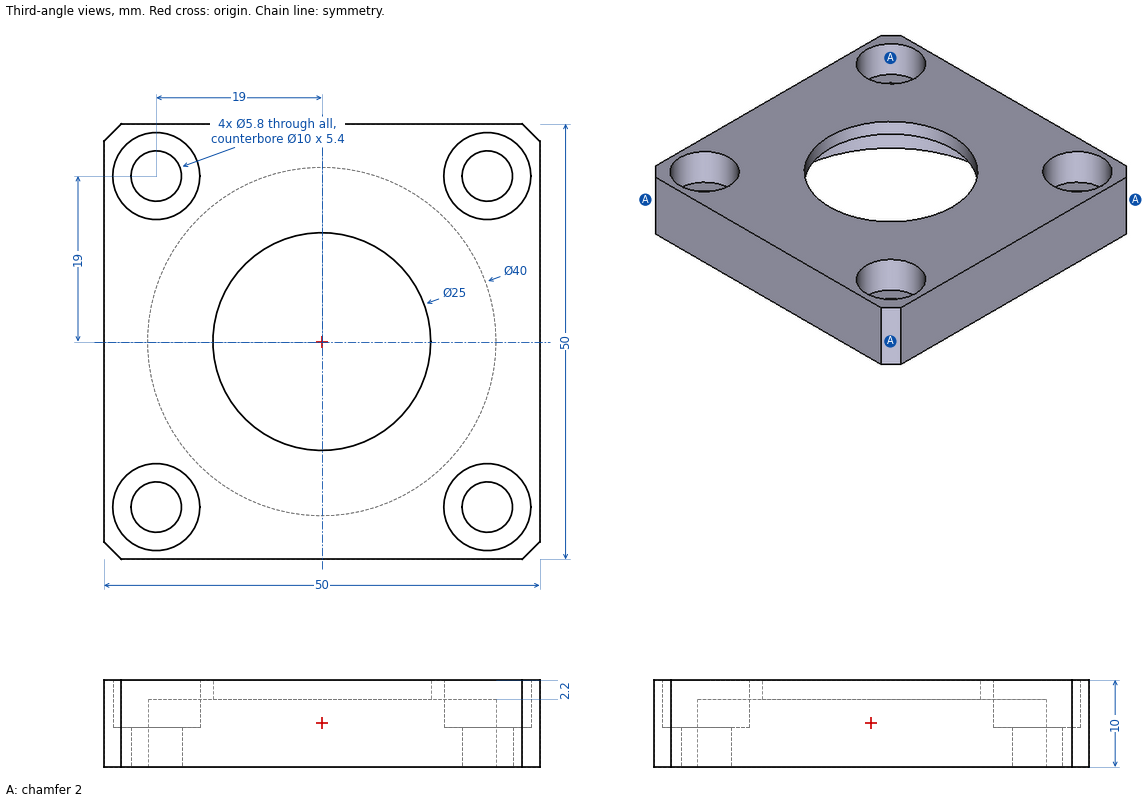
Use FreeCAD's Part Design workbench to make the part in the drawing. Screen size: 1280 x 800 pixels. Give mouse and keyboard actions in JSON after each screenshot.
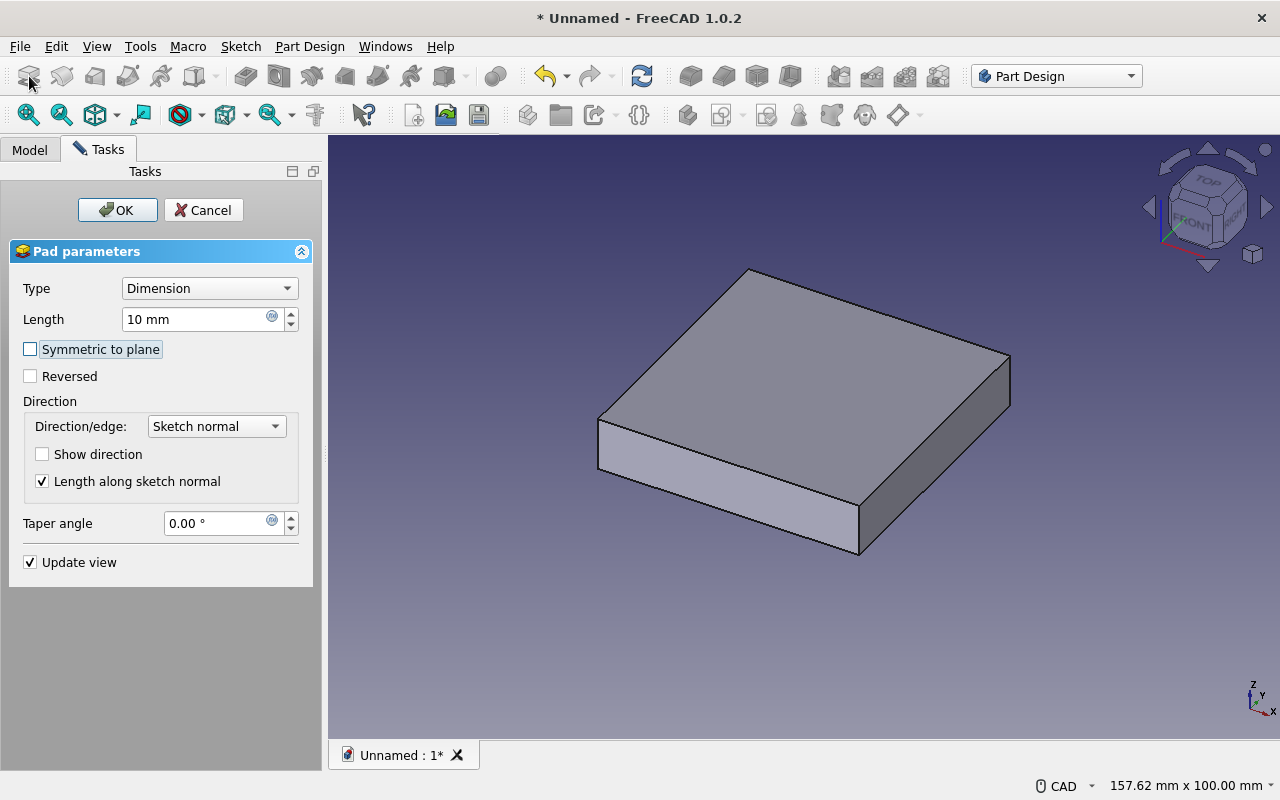
{"action": "left_click", "coordinate": [31, 349]}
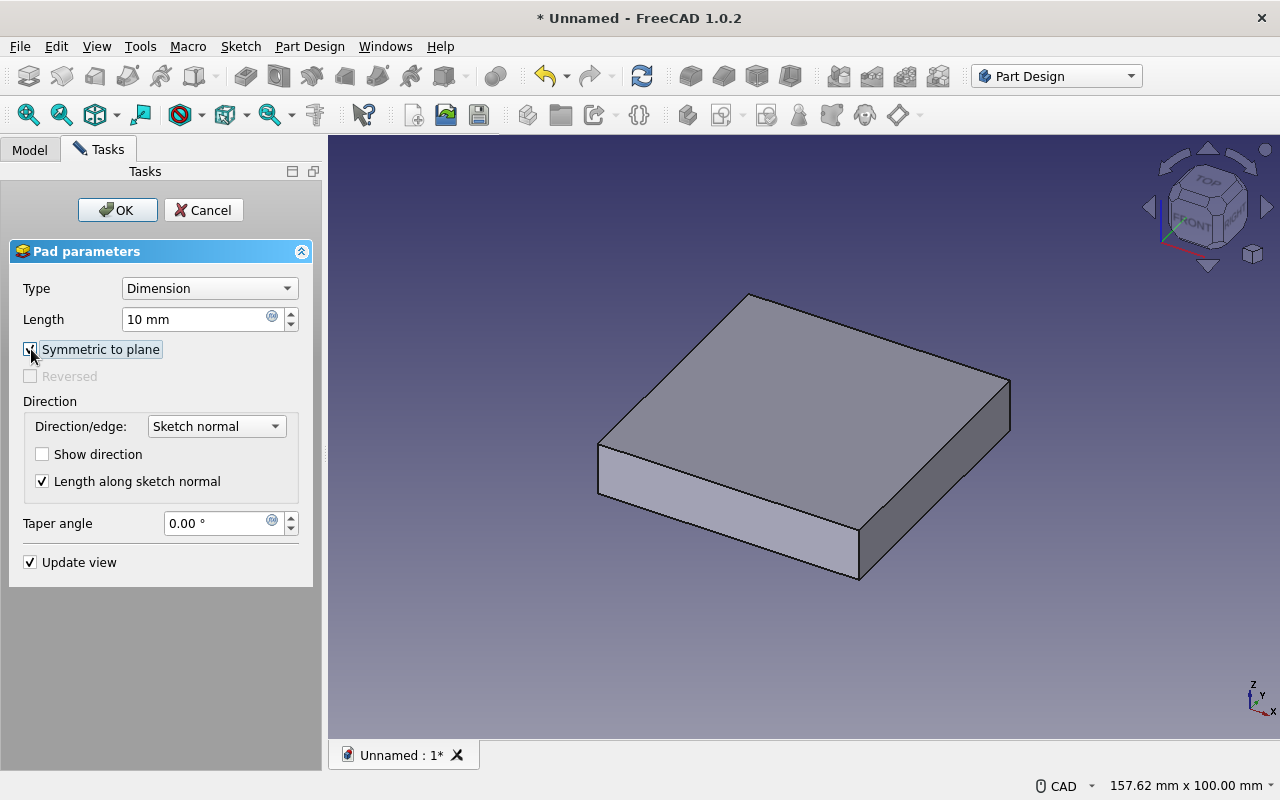
{"action": "left_click", "coordinate": [118, 210]}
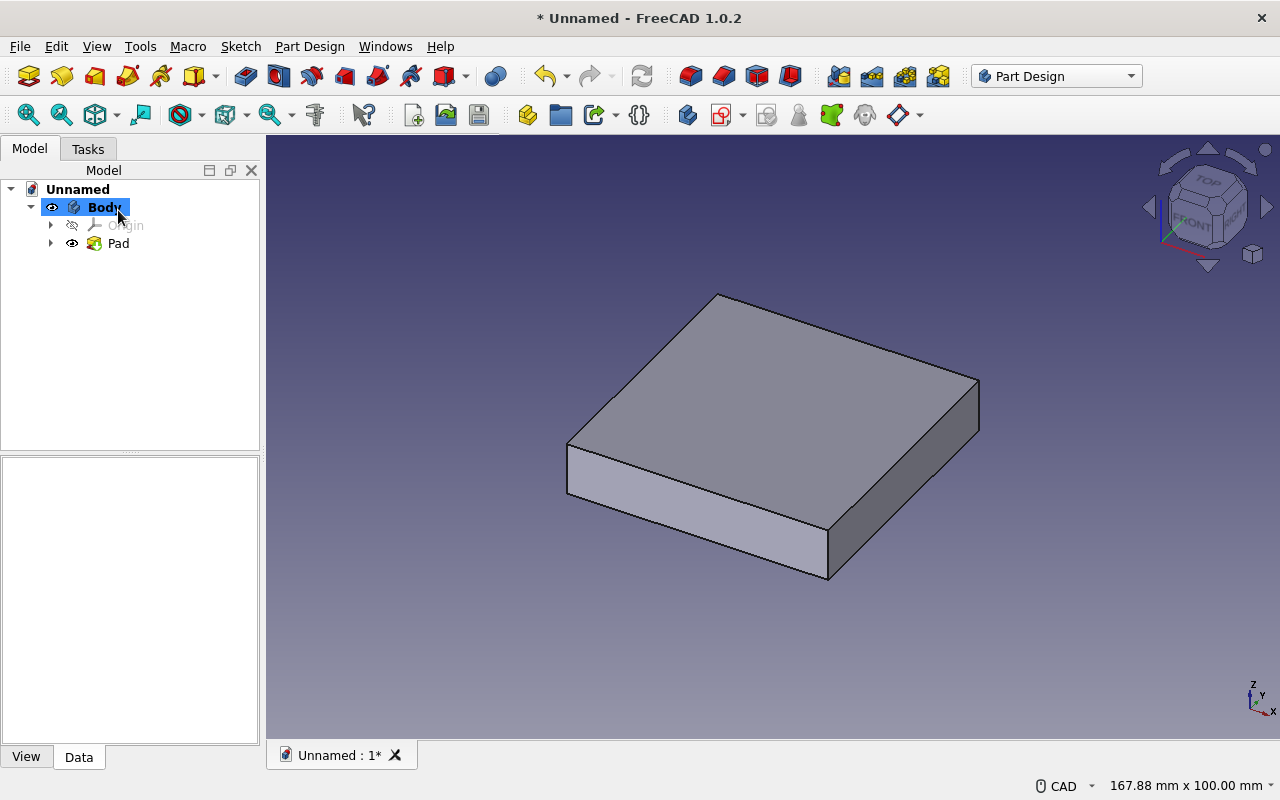
{"action": "left_click", "coordinate": [773, 411]}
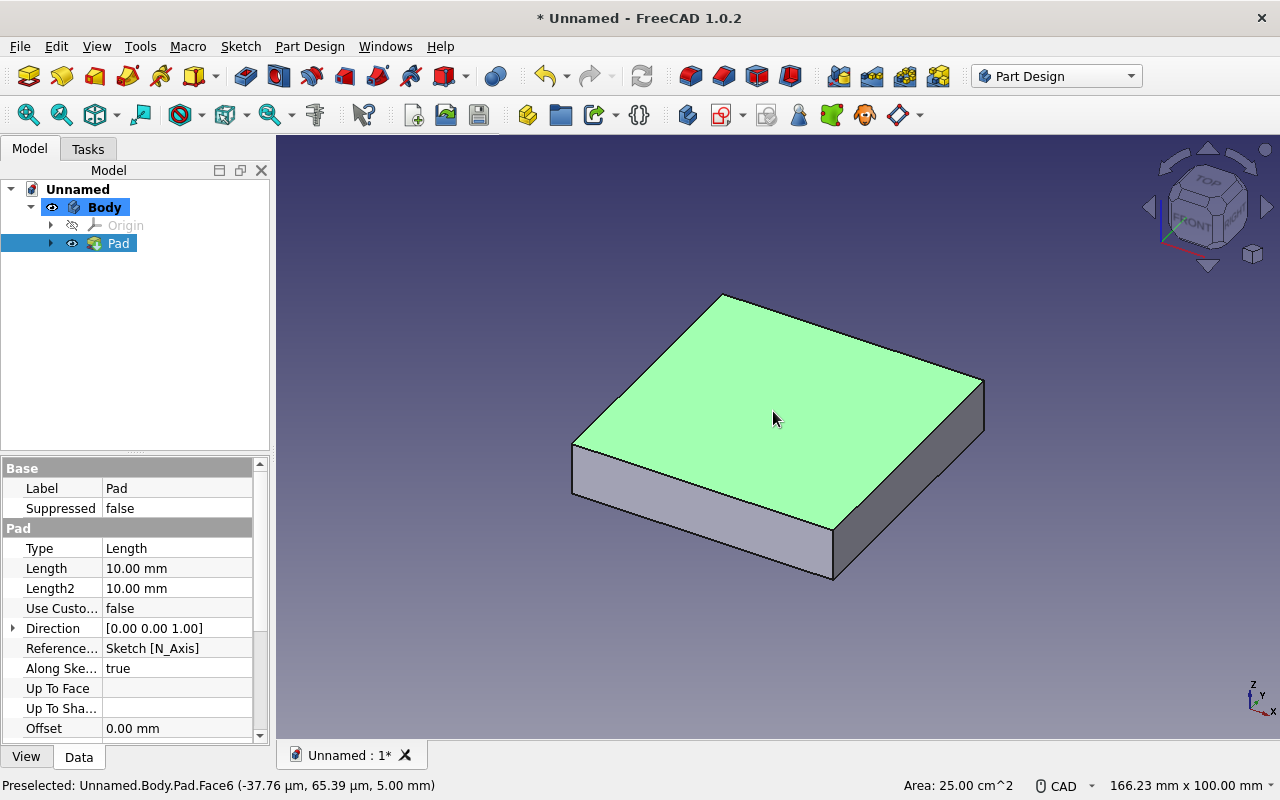
{"action": "left_click", "coordinate": [720, 116]}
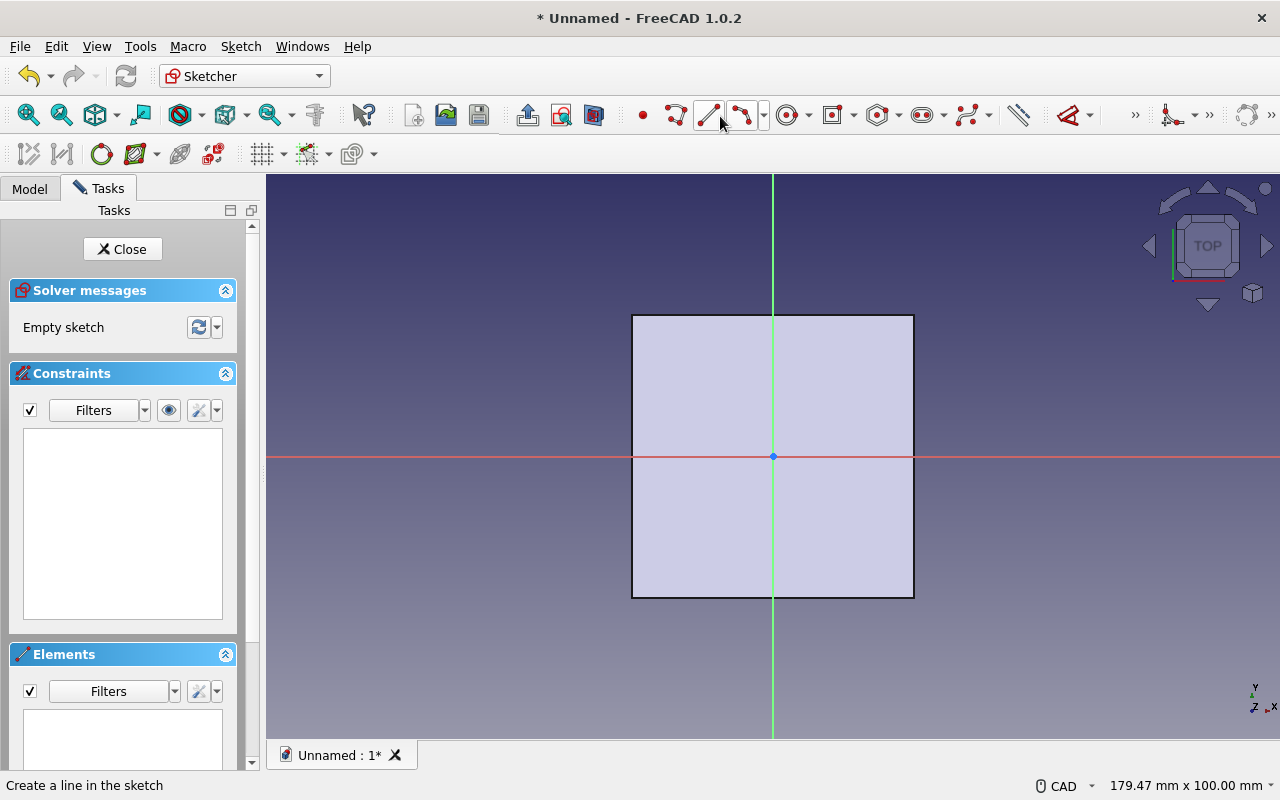
{"action": "scroll", "coordinate": [912, 456], "scroll_direction": "up", "scroll_amount": 2}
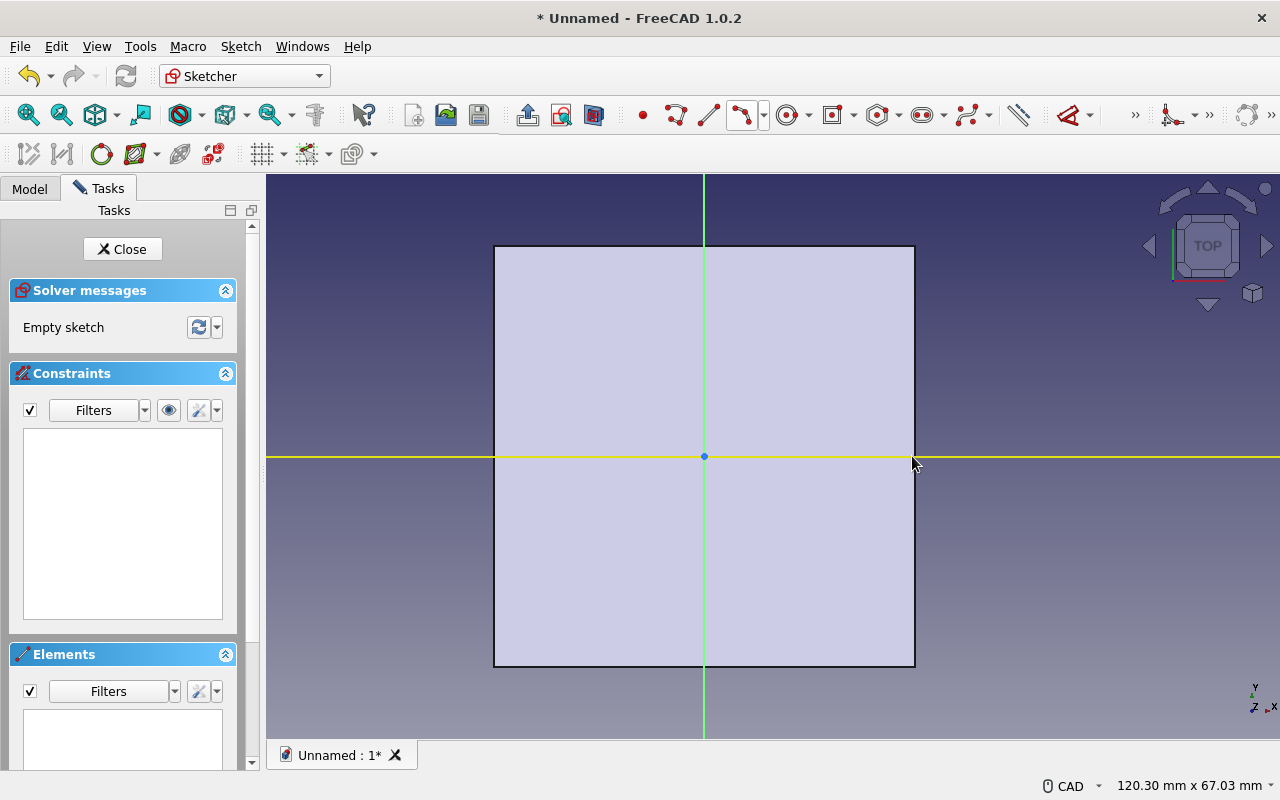
{"action": "left_click", "coordinate": [786, 116]}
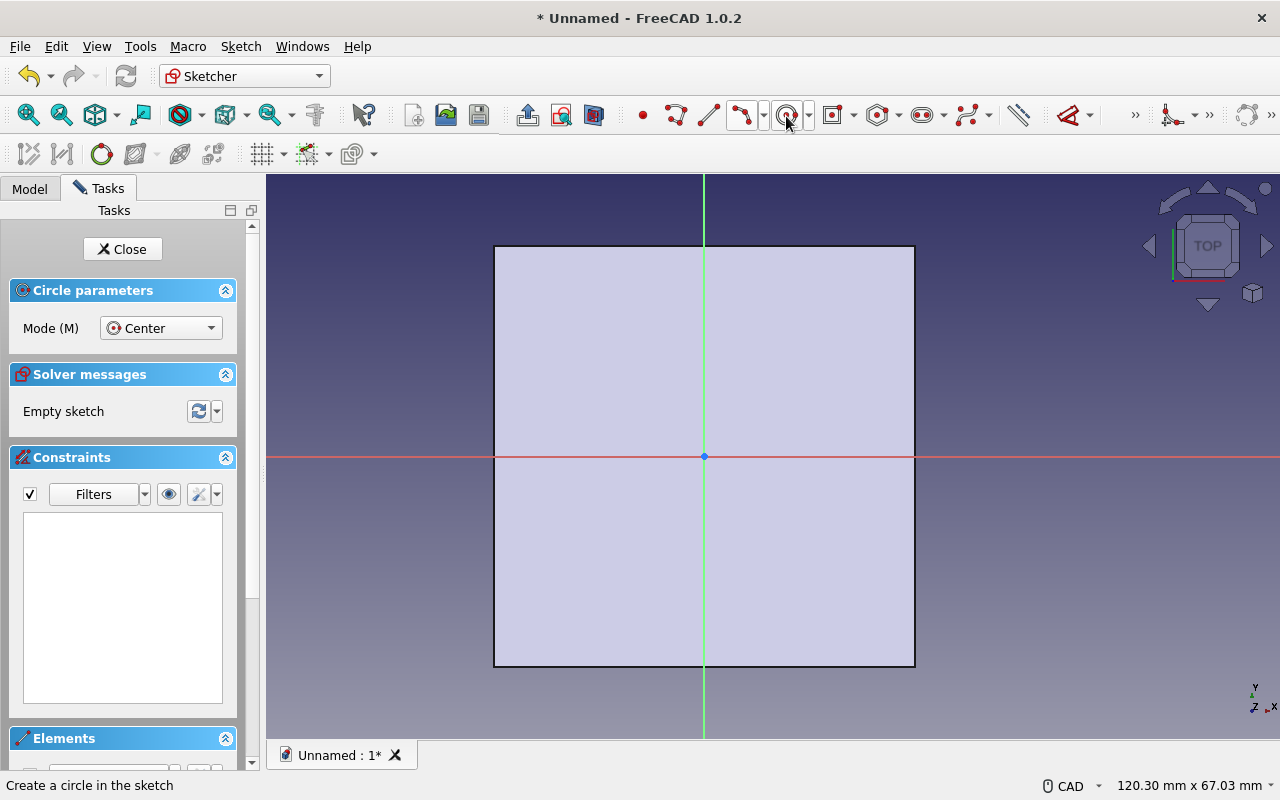
{"action": "left_click", "coordinate": [704, 456]}
{"action": "mouse_move", "coordinate": [824, 337]}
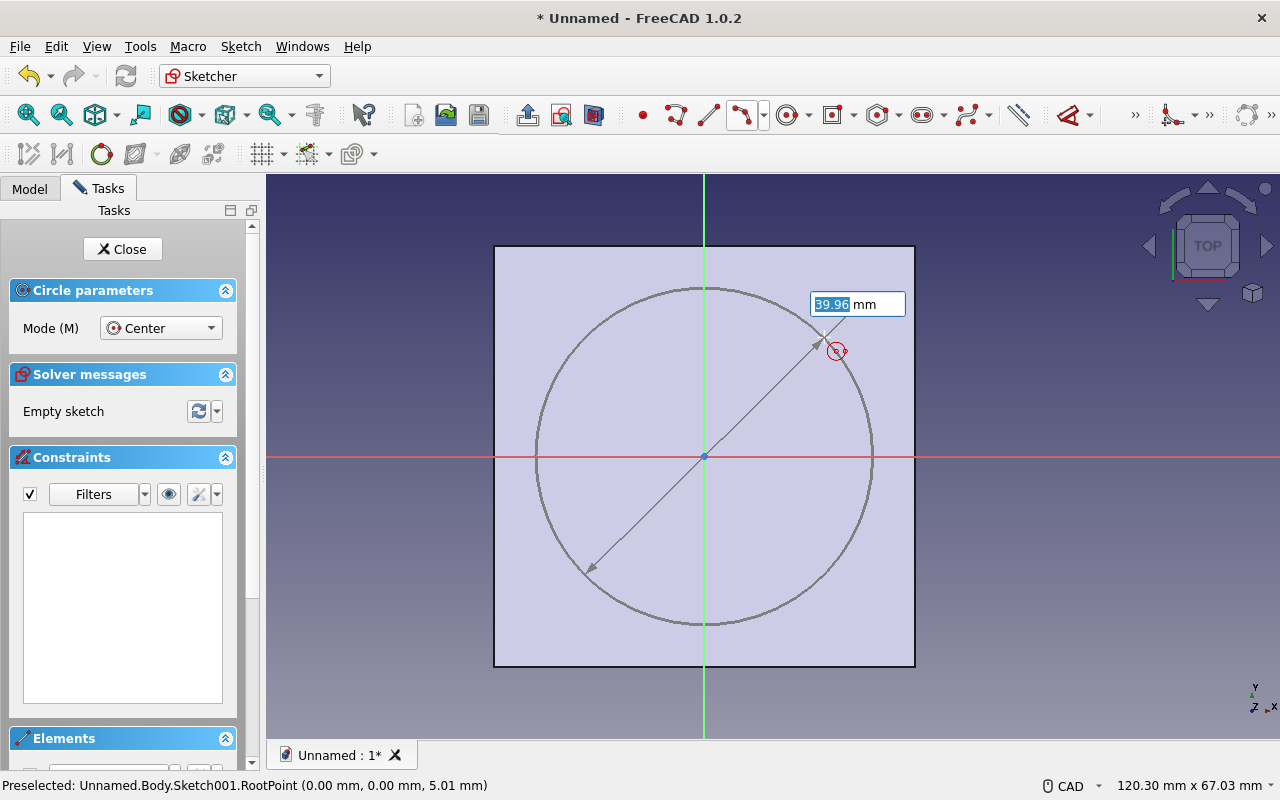
{"action": "type", "text": "40"}
{"action": "key", "text": "Return"}
{"action": "key", "text": "Escape"}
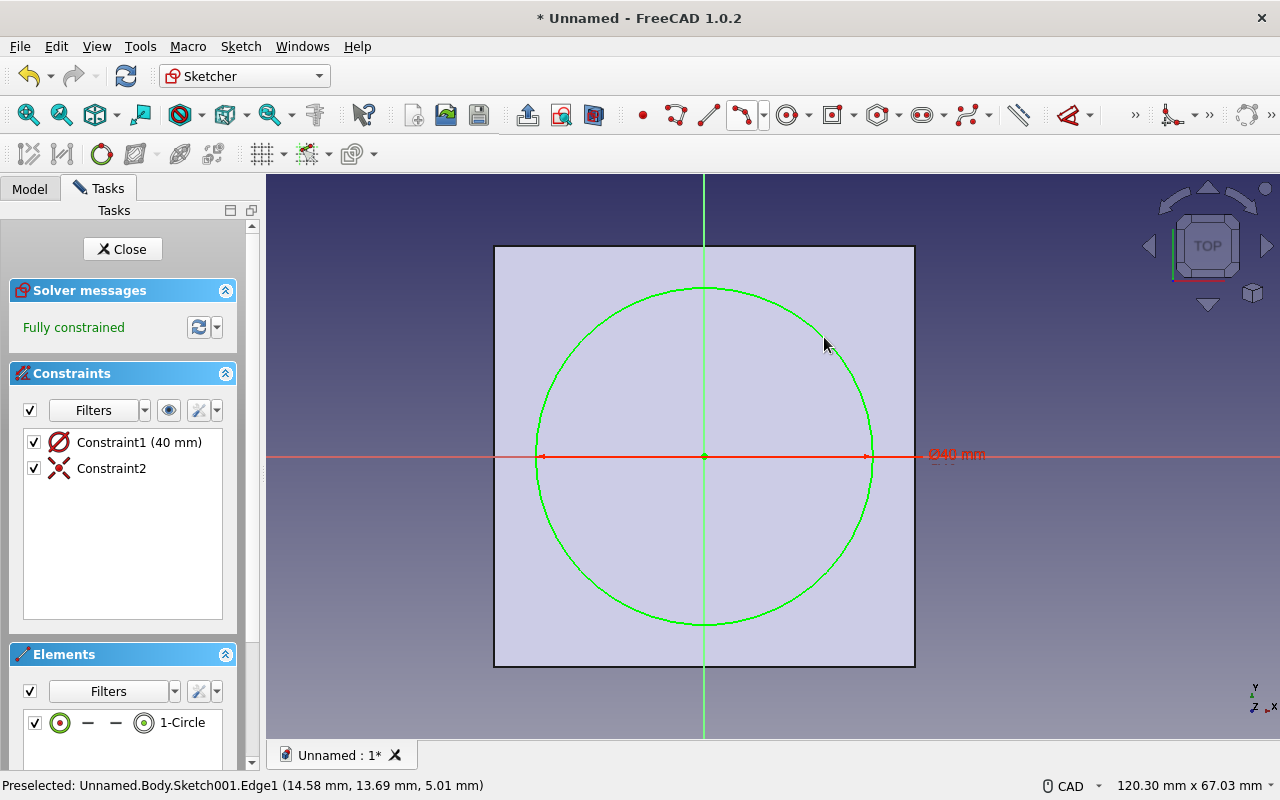
{"action": "left_click", "coordinate": [123, 249]}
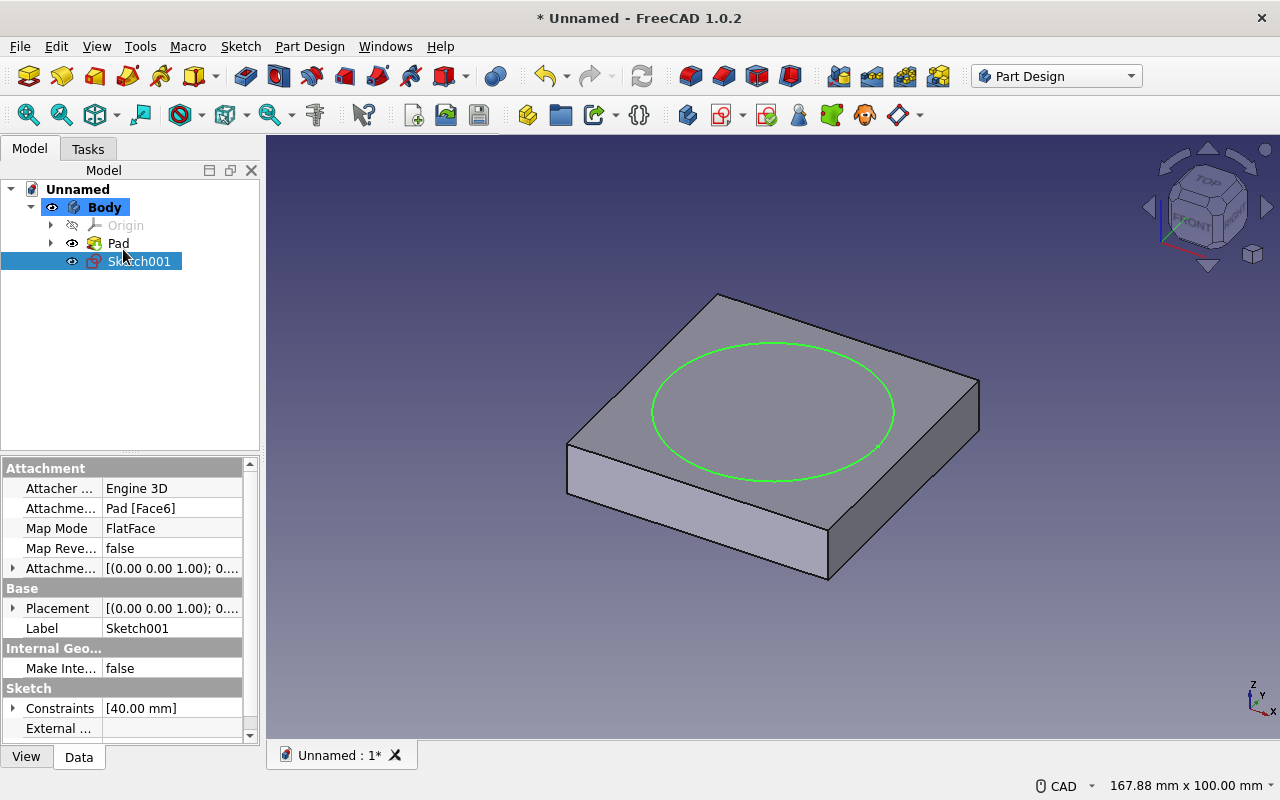
{"action": "left_click", "coordinate": [246, 76]}